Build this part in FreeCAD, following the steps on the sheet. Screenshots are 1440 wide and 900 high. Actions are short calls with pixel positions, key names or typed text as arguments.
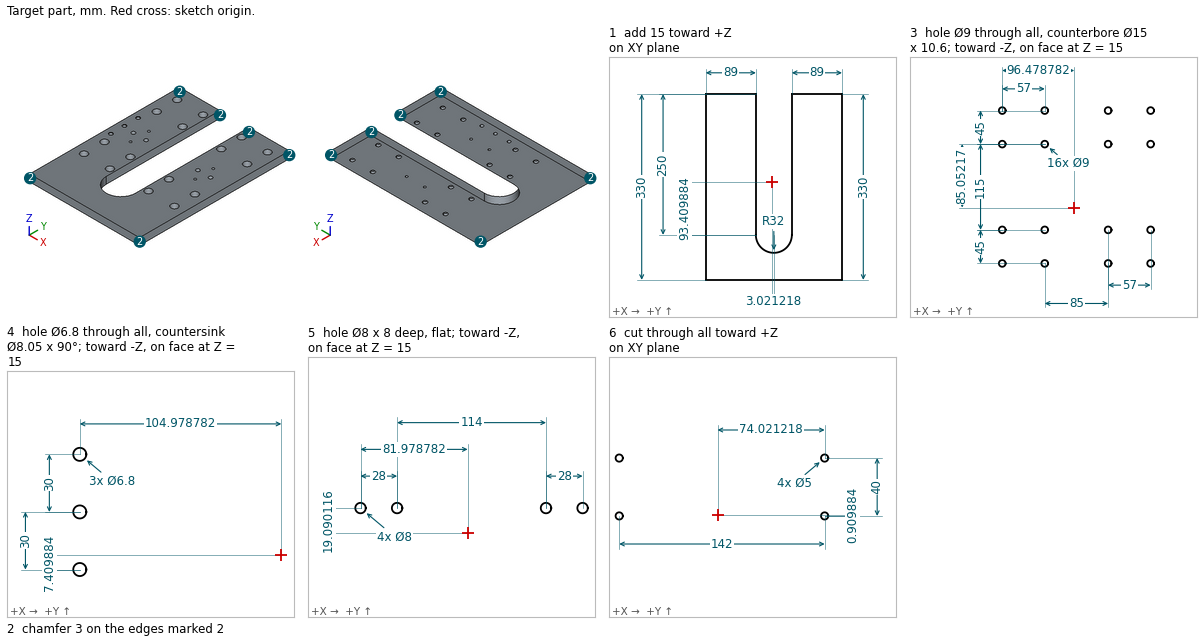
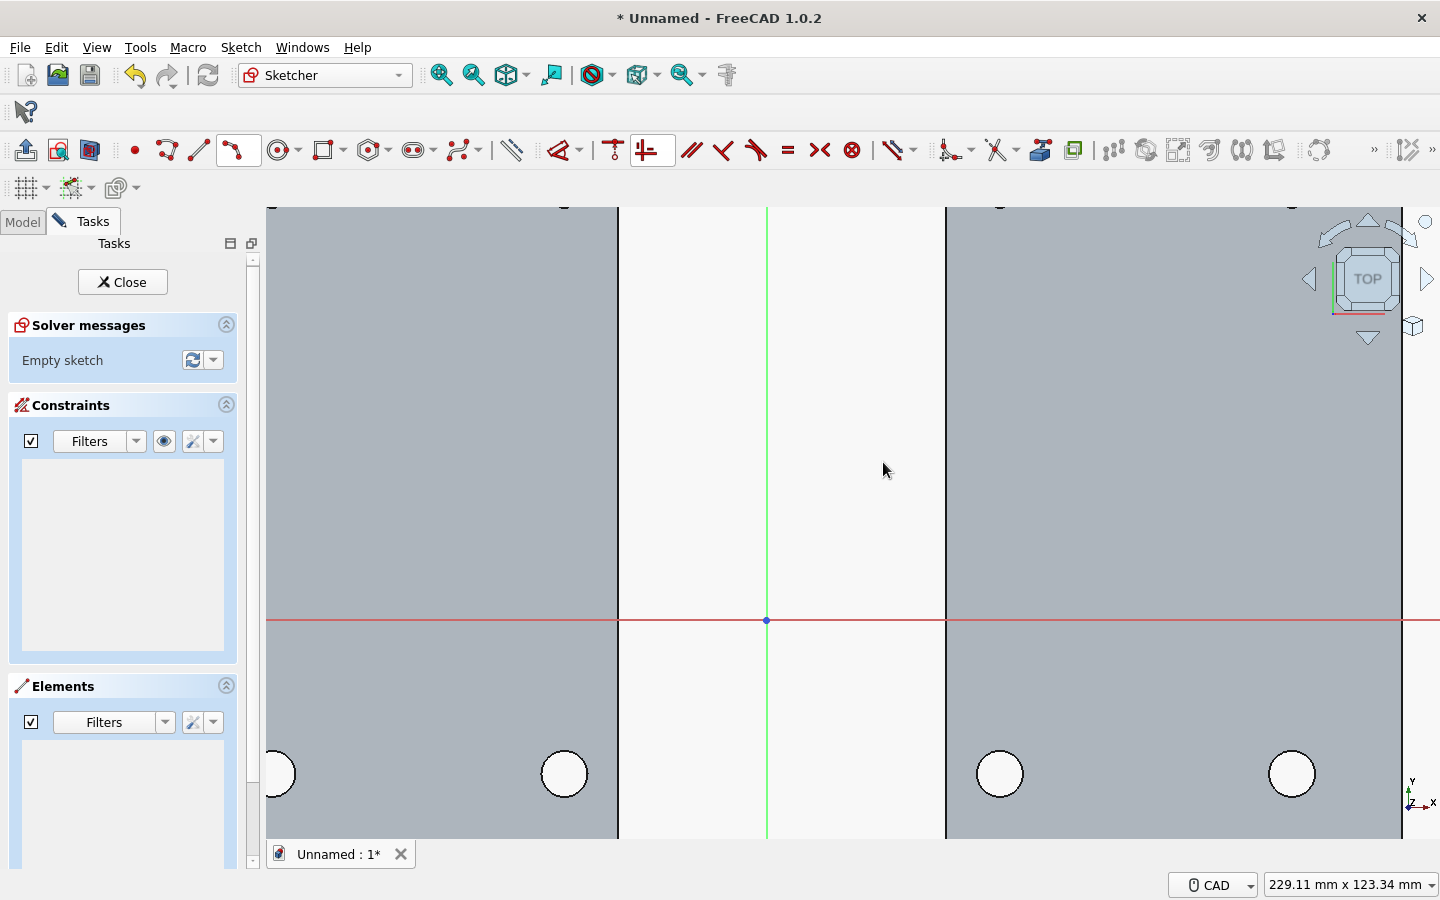
key(g)
key(c)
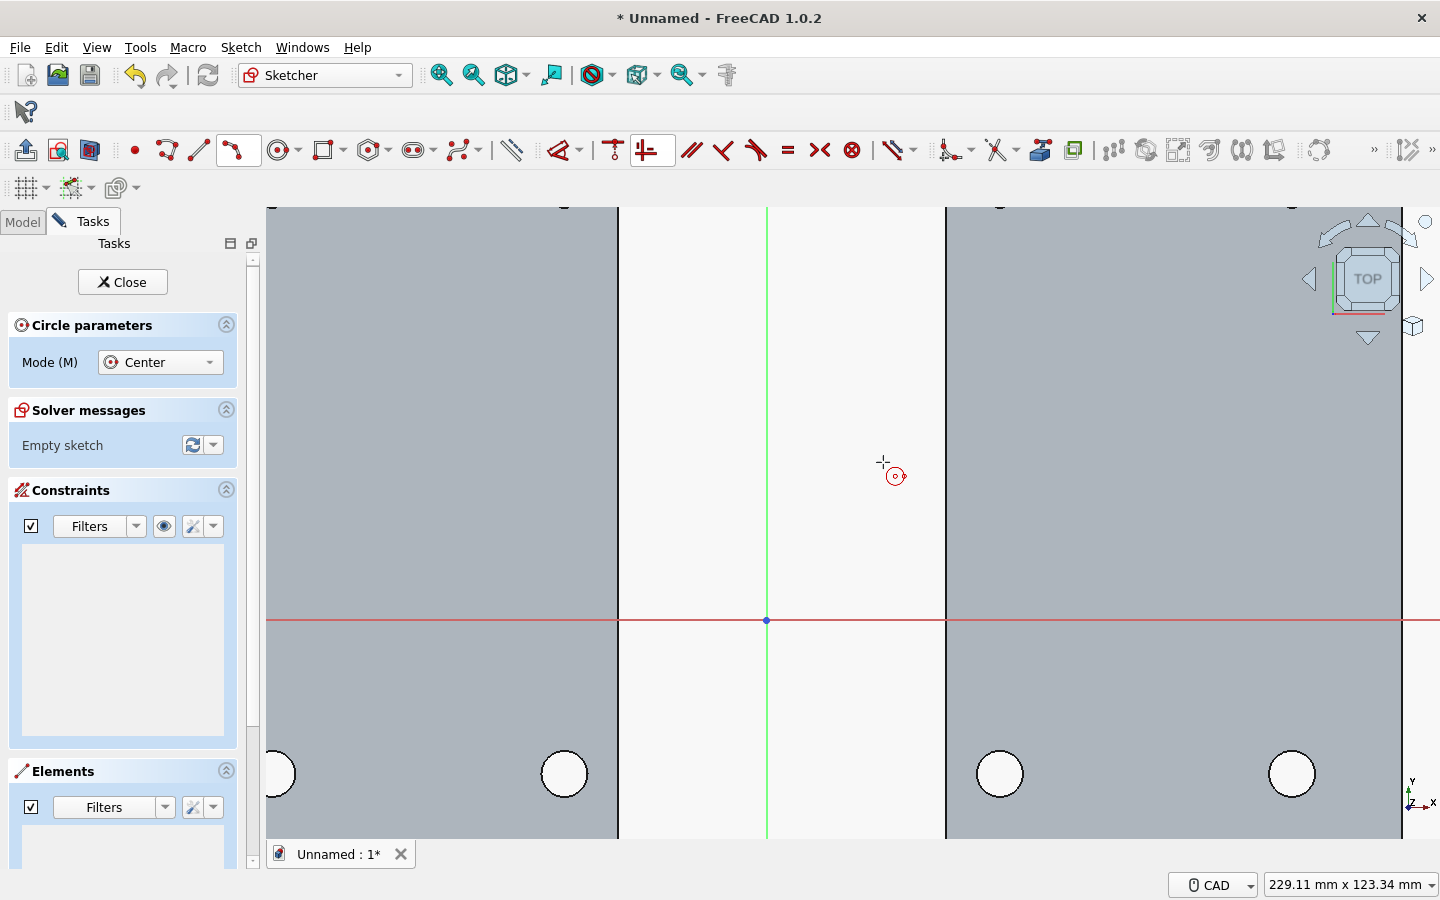
scroll(1146, 420, up, 3)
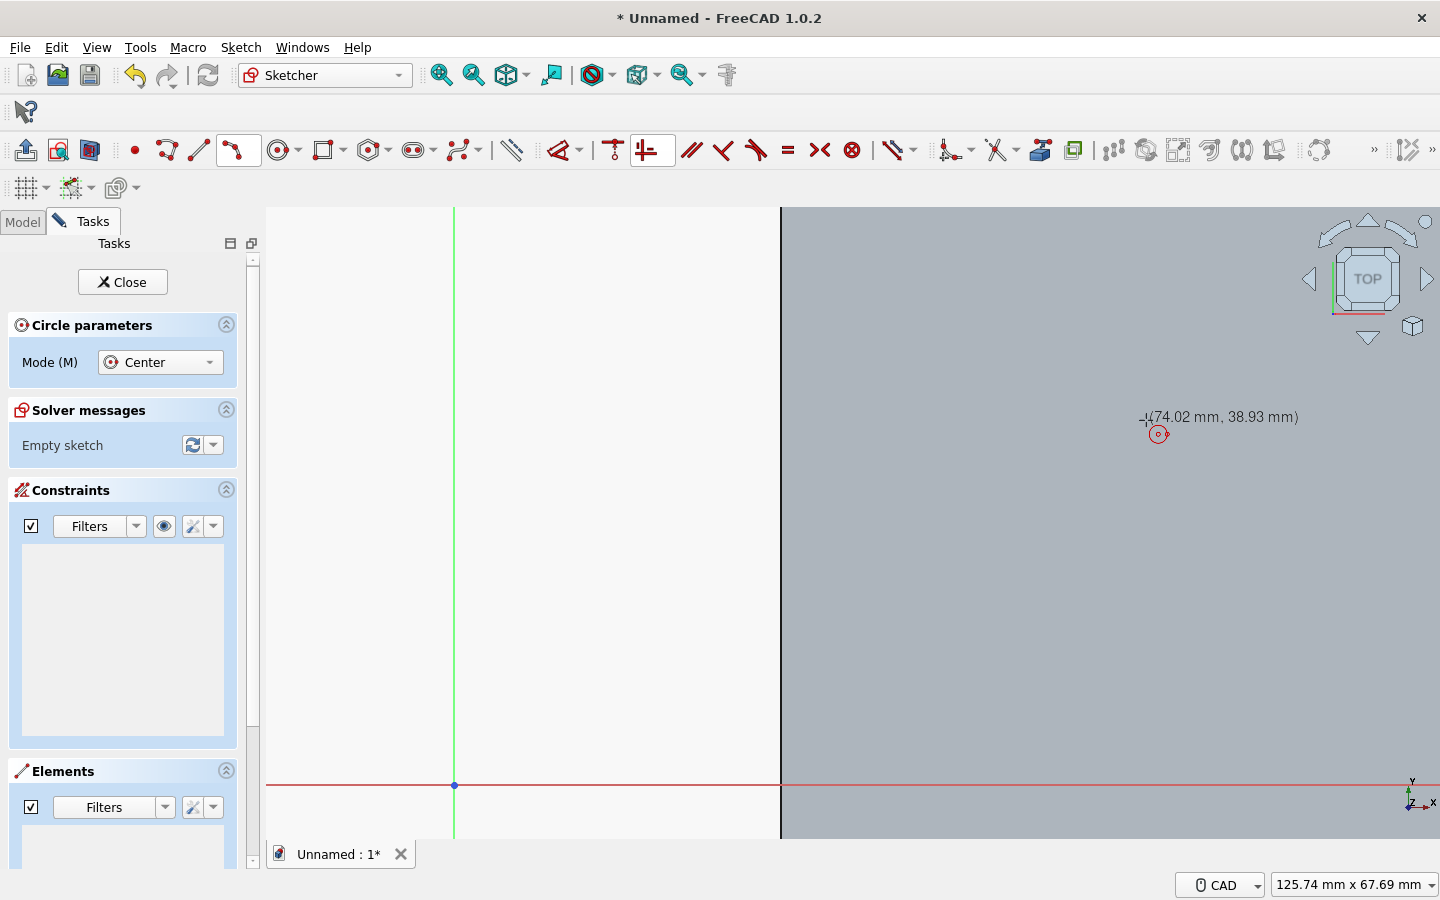
click(1145, 420)
move(1162, 404)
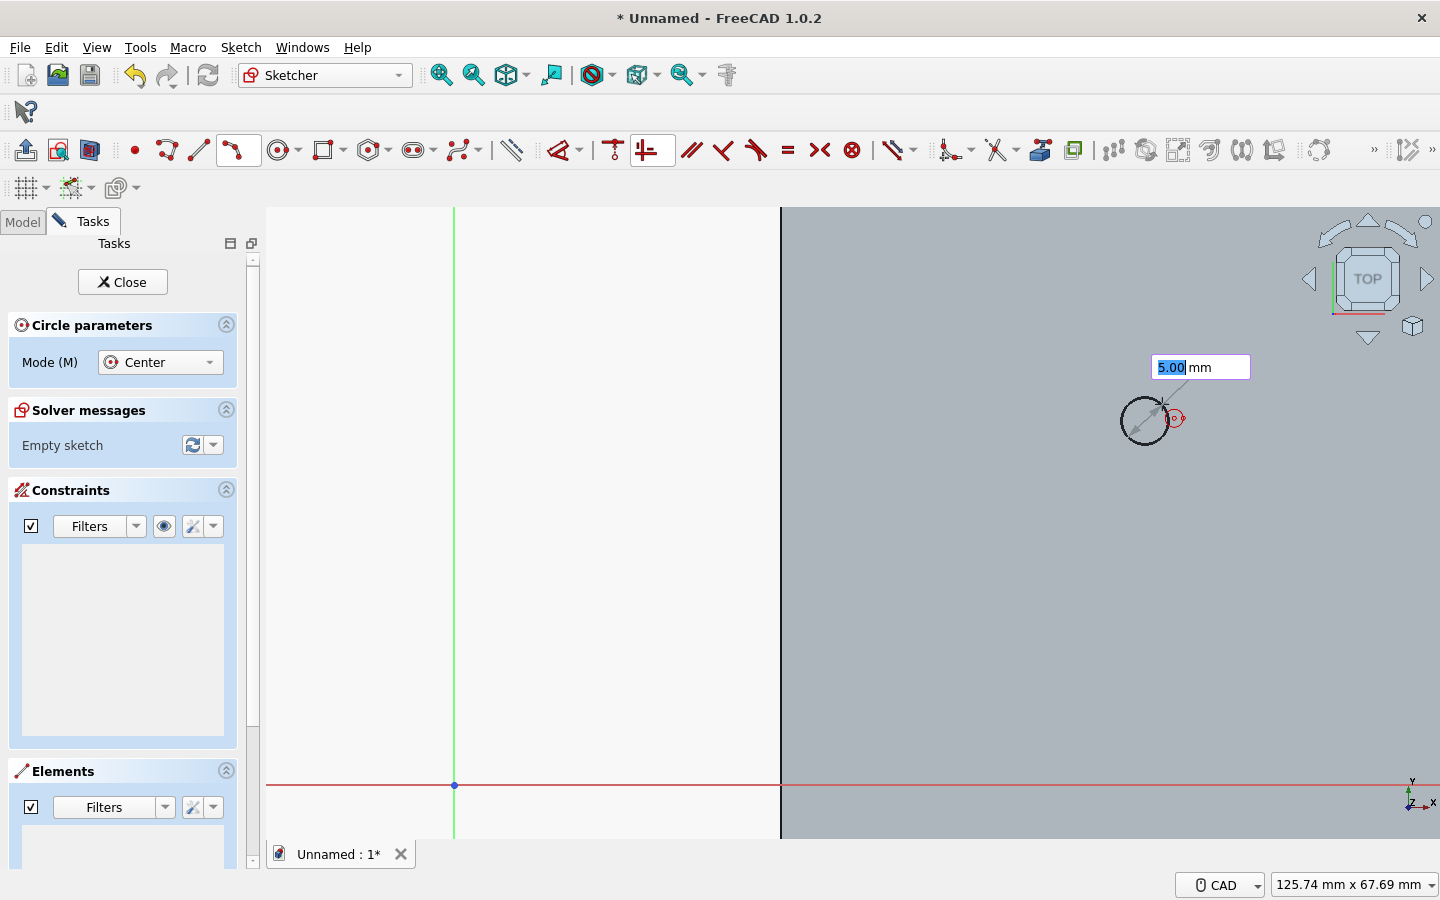
text(5)
key(Return)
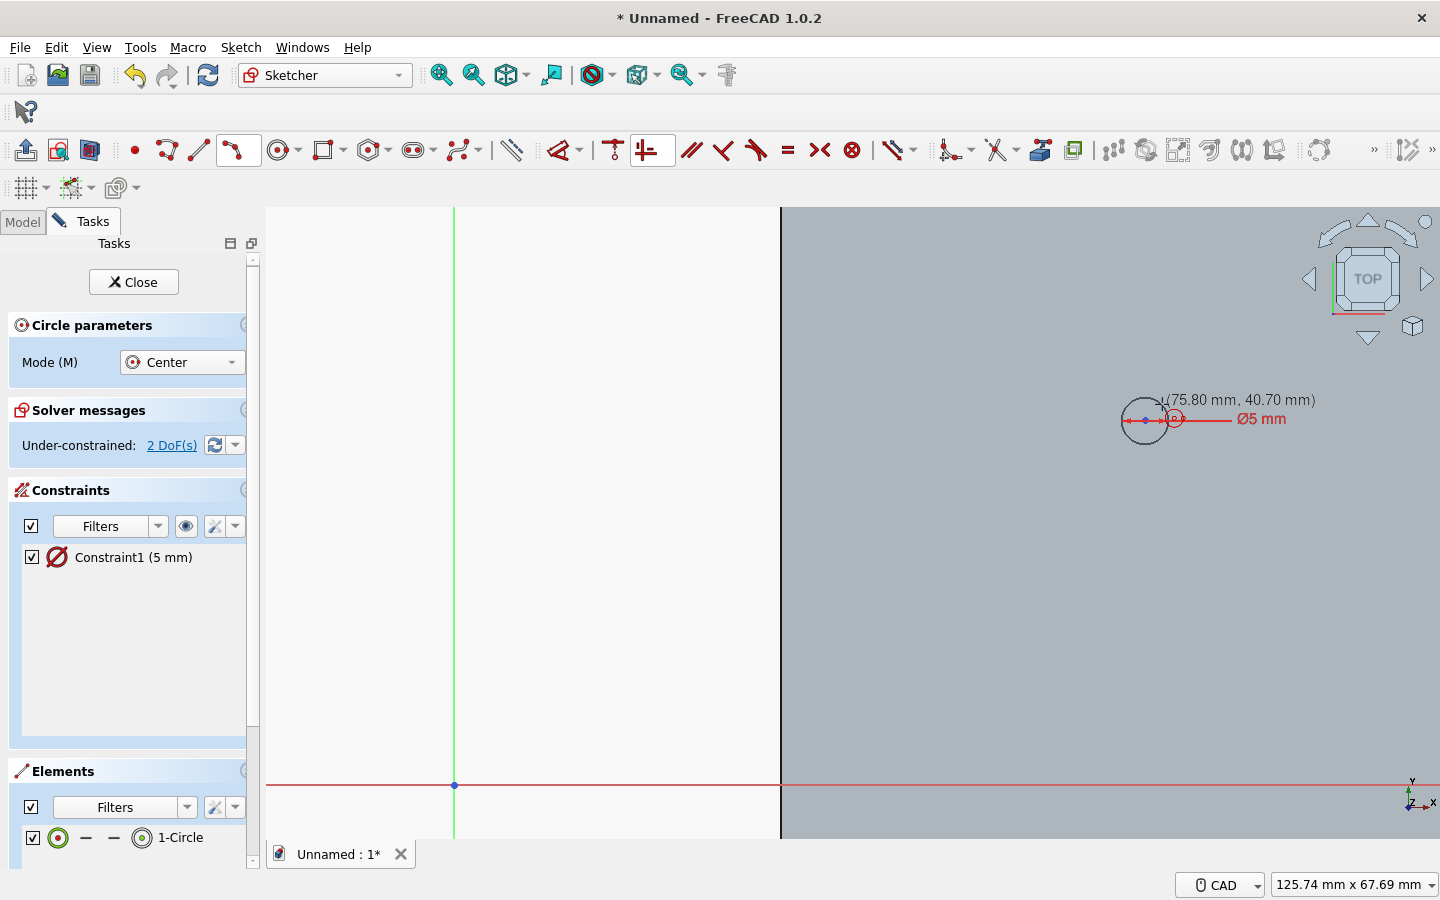
scroll(1145, 794, up, 4)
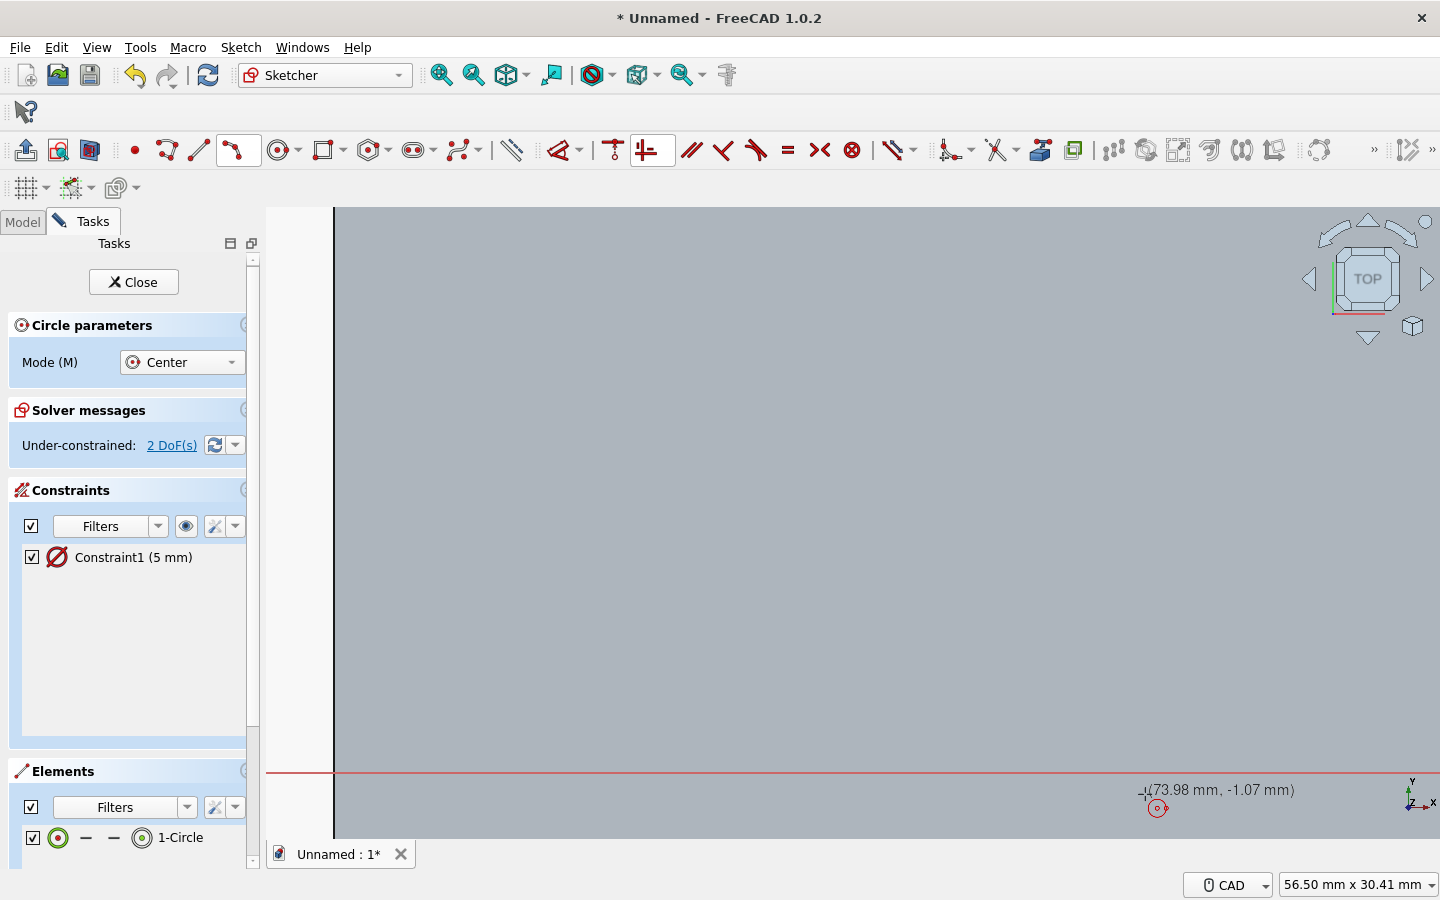
click(1145, 792)
move(1182, 755)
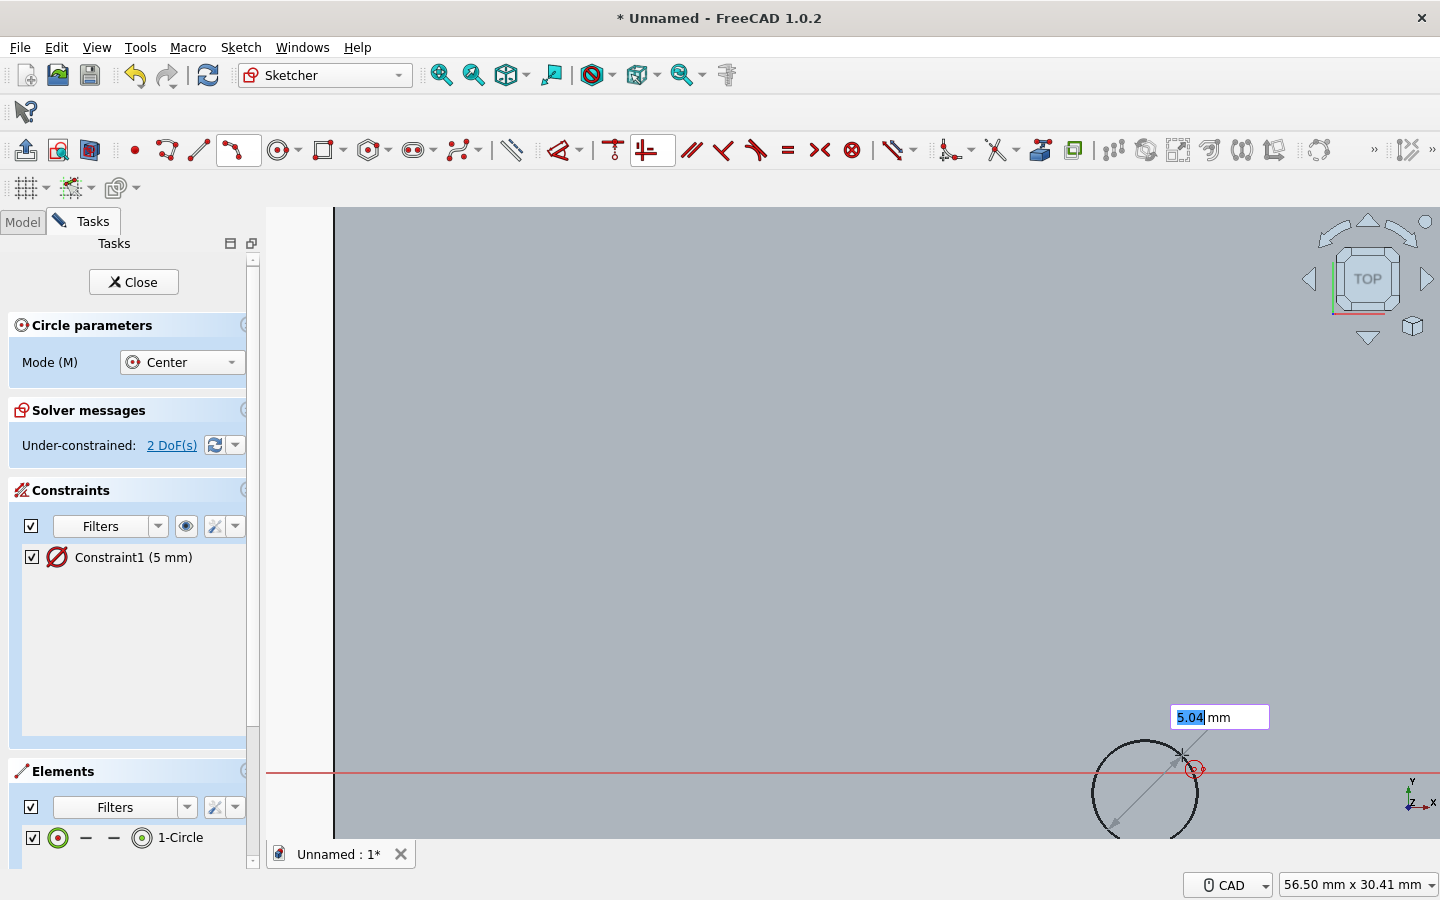
text(5)
key(Return)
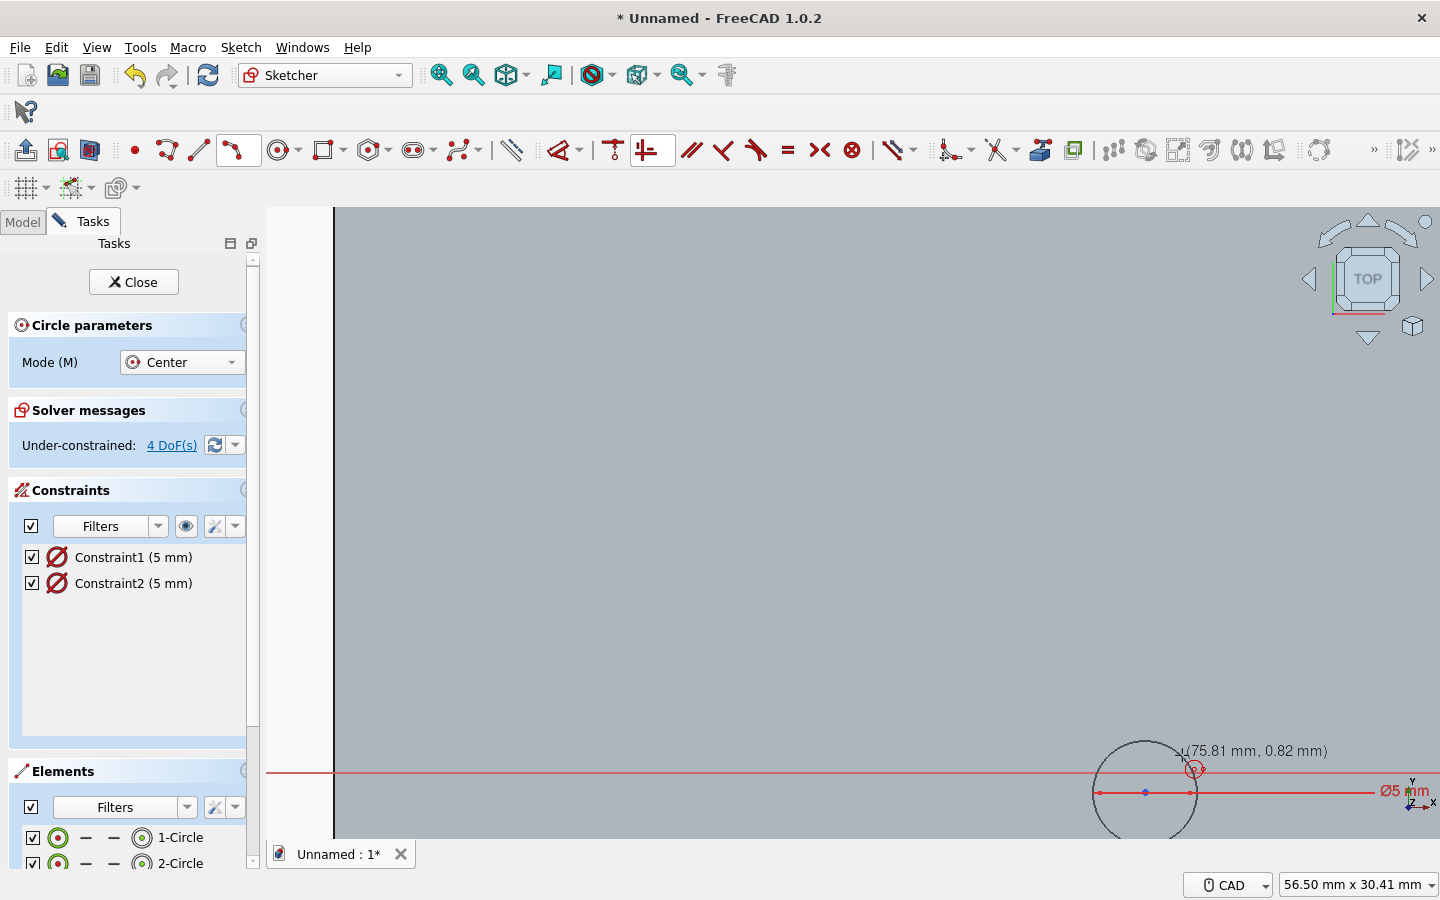
scroll(1149, 571, down, 7)